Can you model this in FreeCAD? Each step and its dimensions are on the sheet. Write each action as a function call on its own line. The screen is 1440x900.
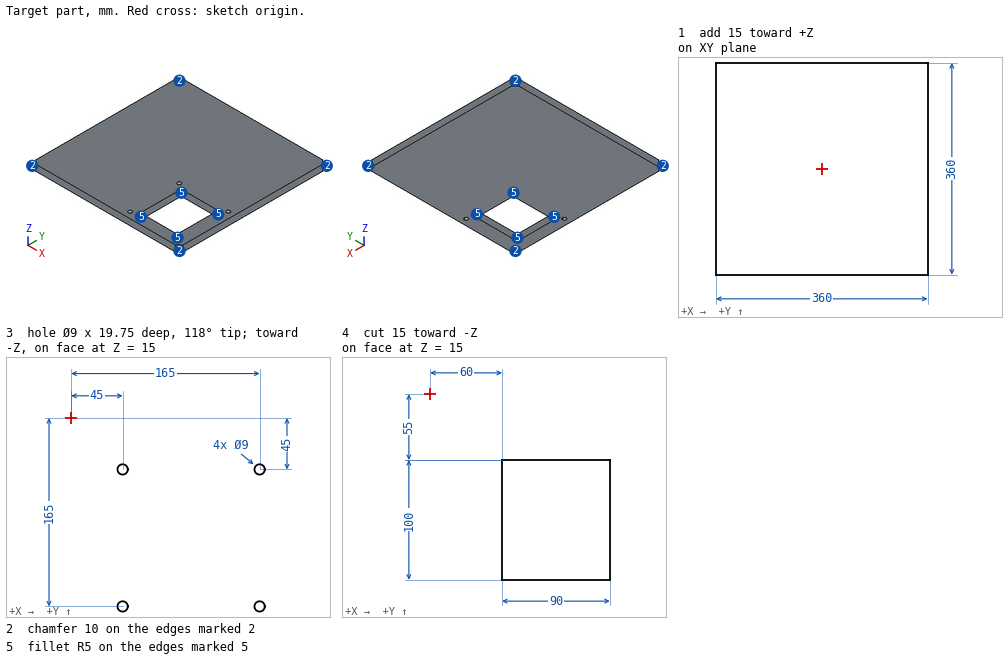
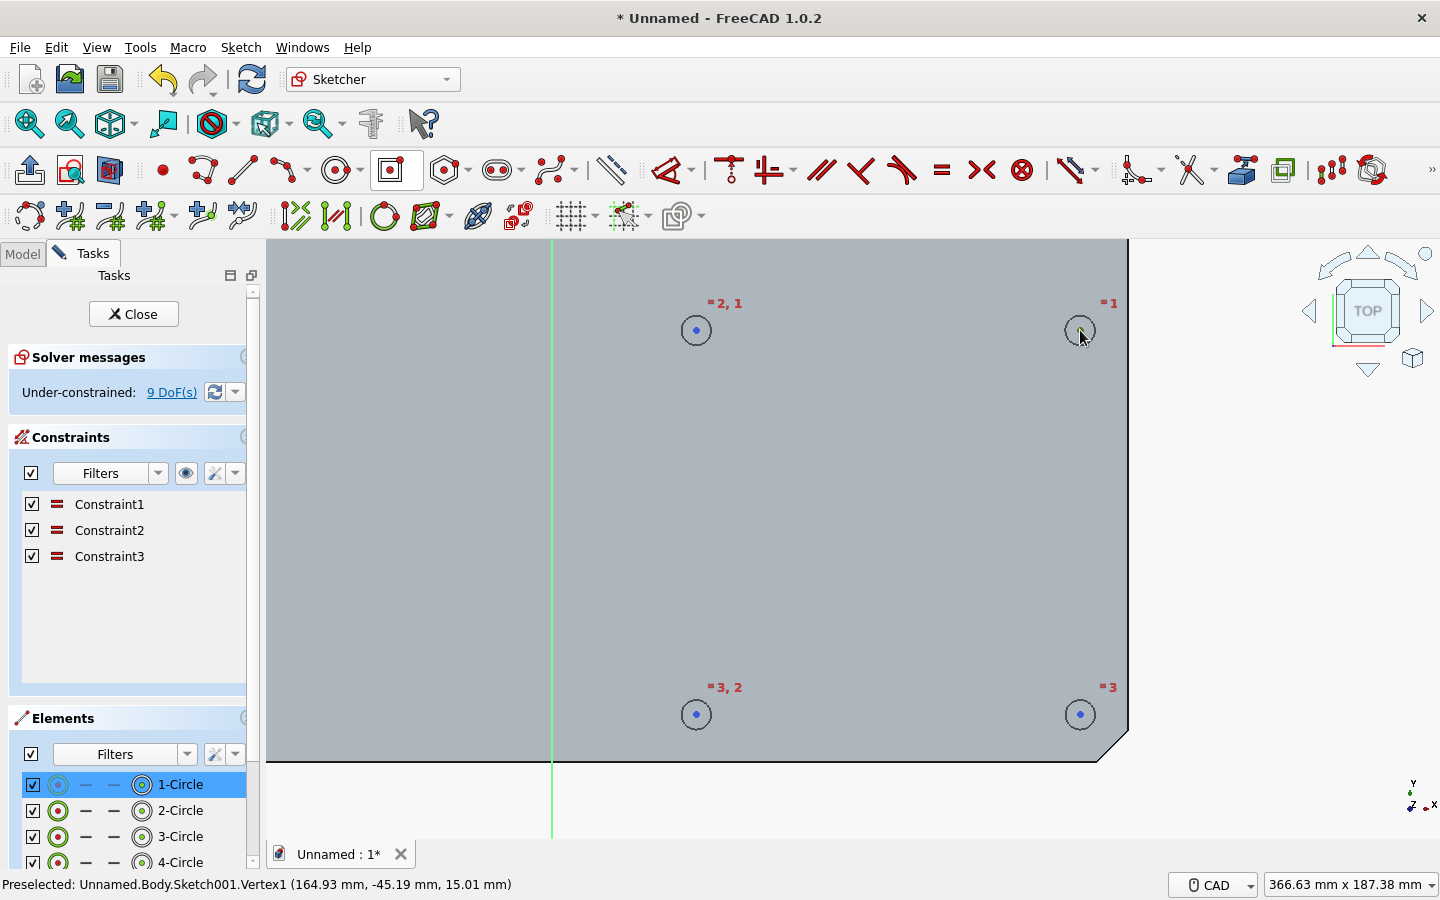
click(696, 330)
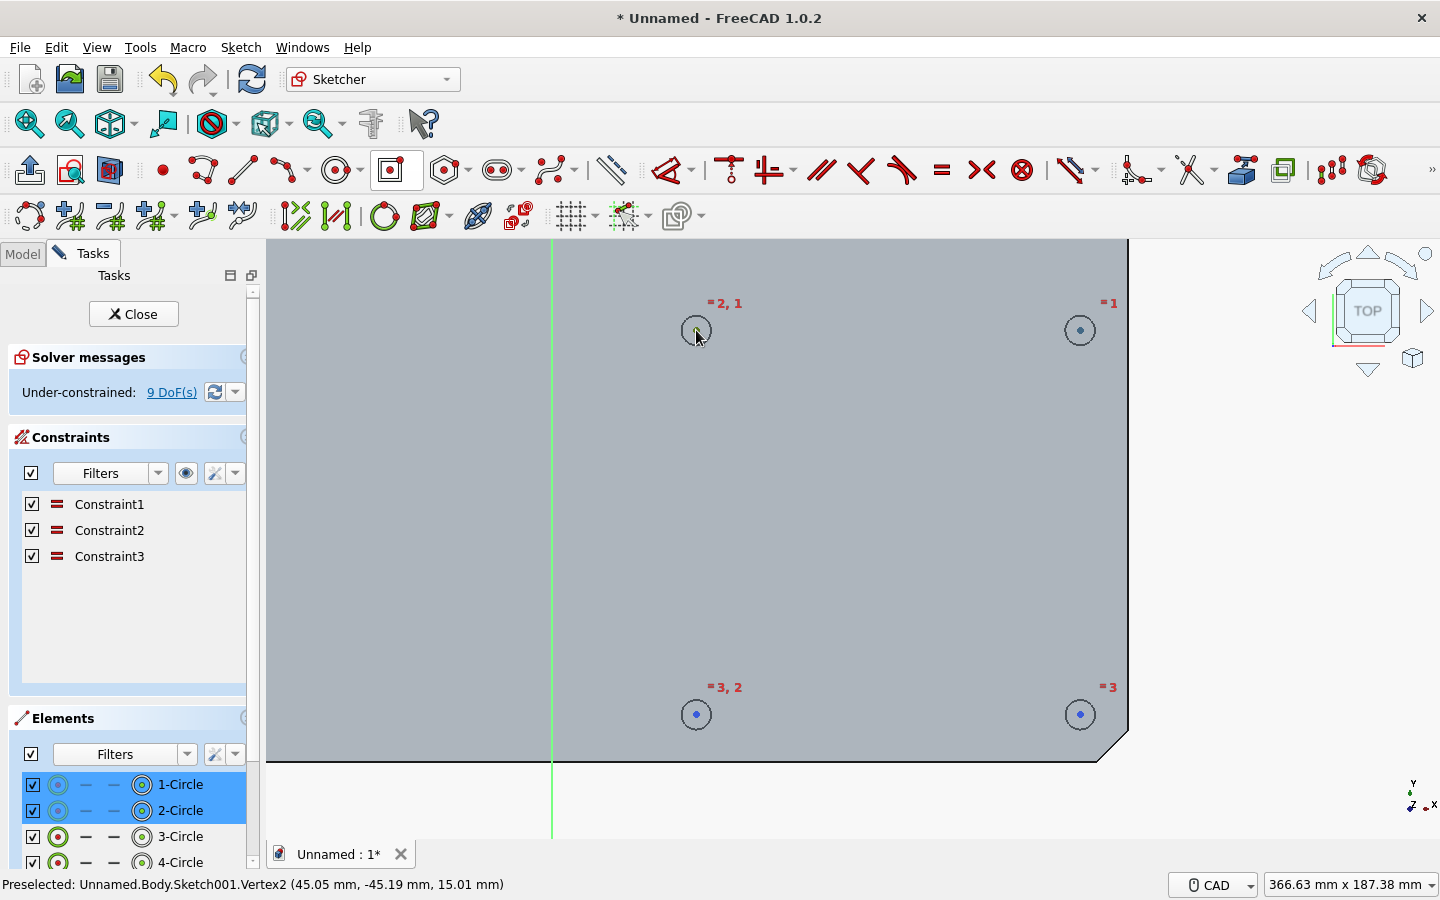
key(h)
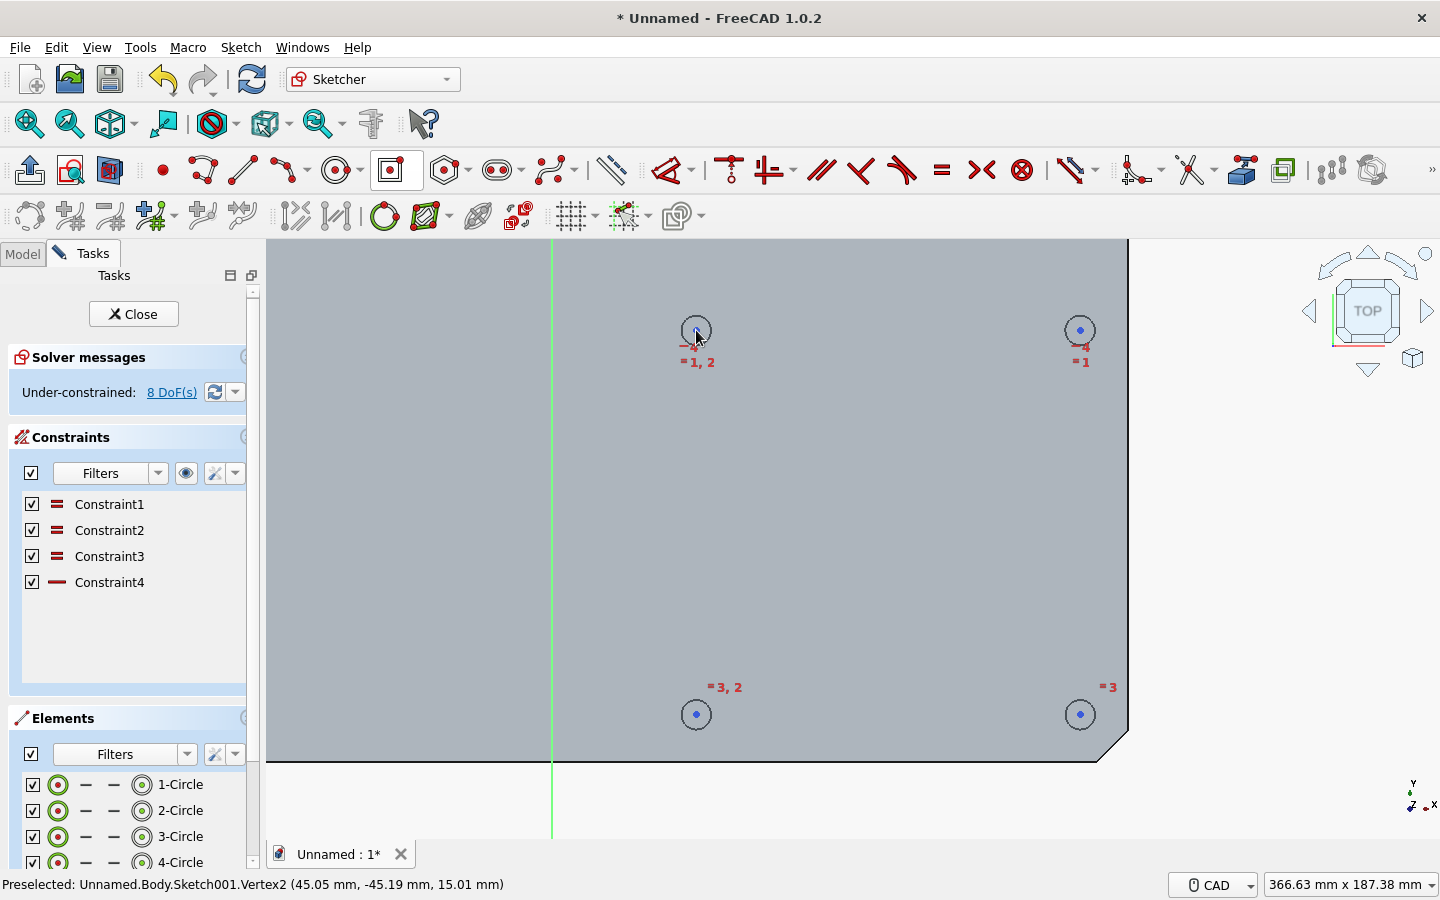
click(696, 330)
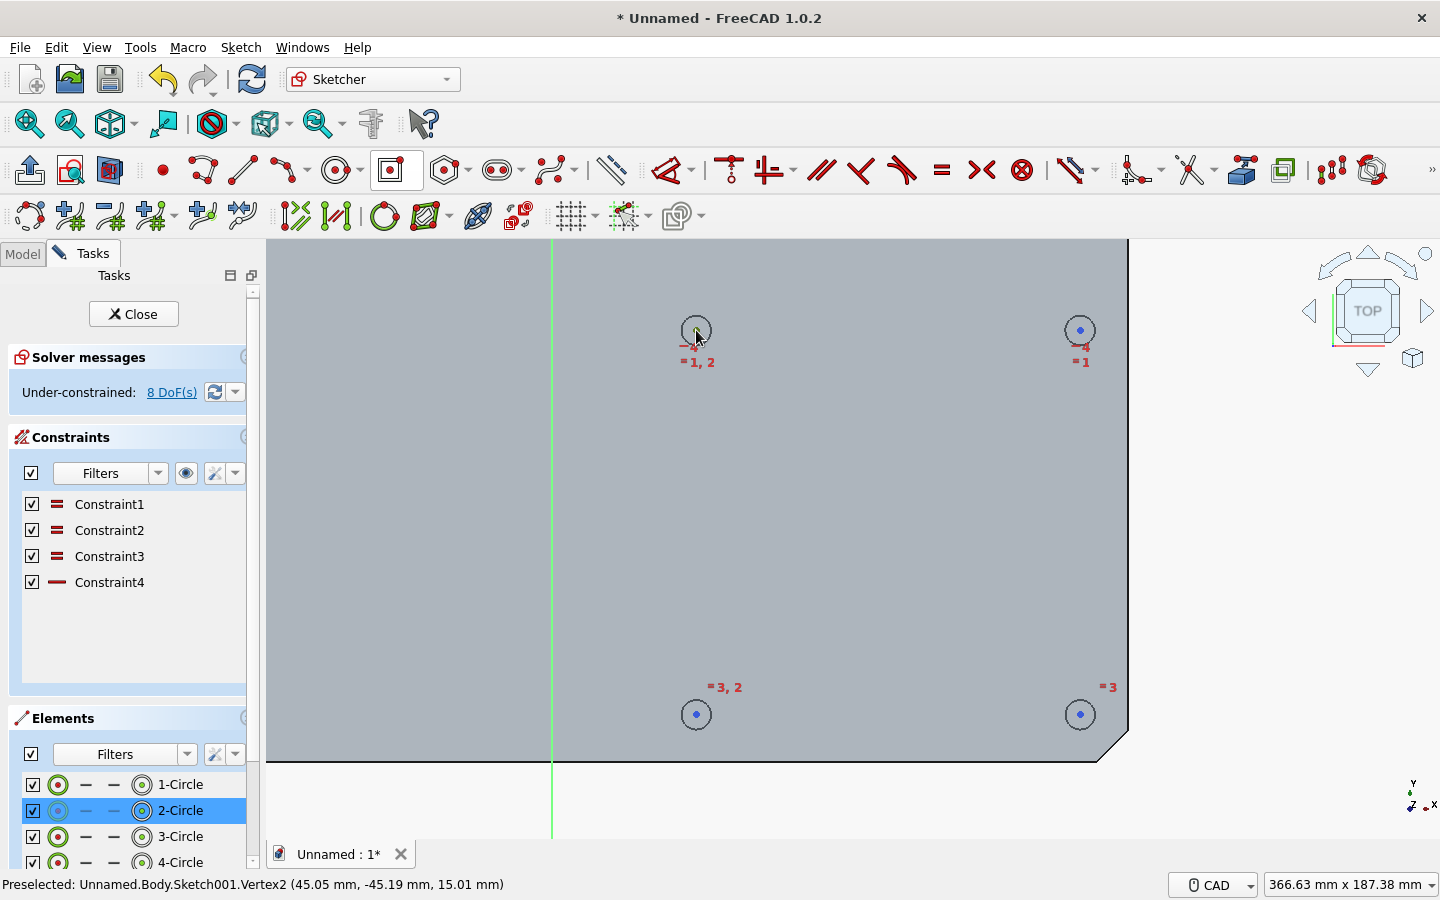
click(696, 715)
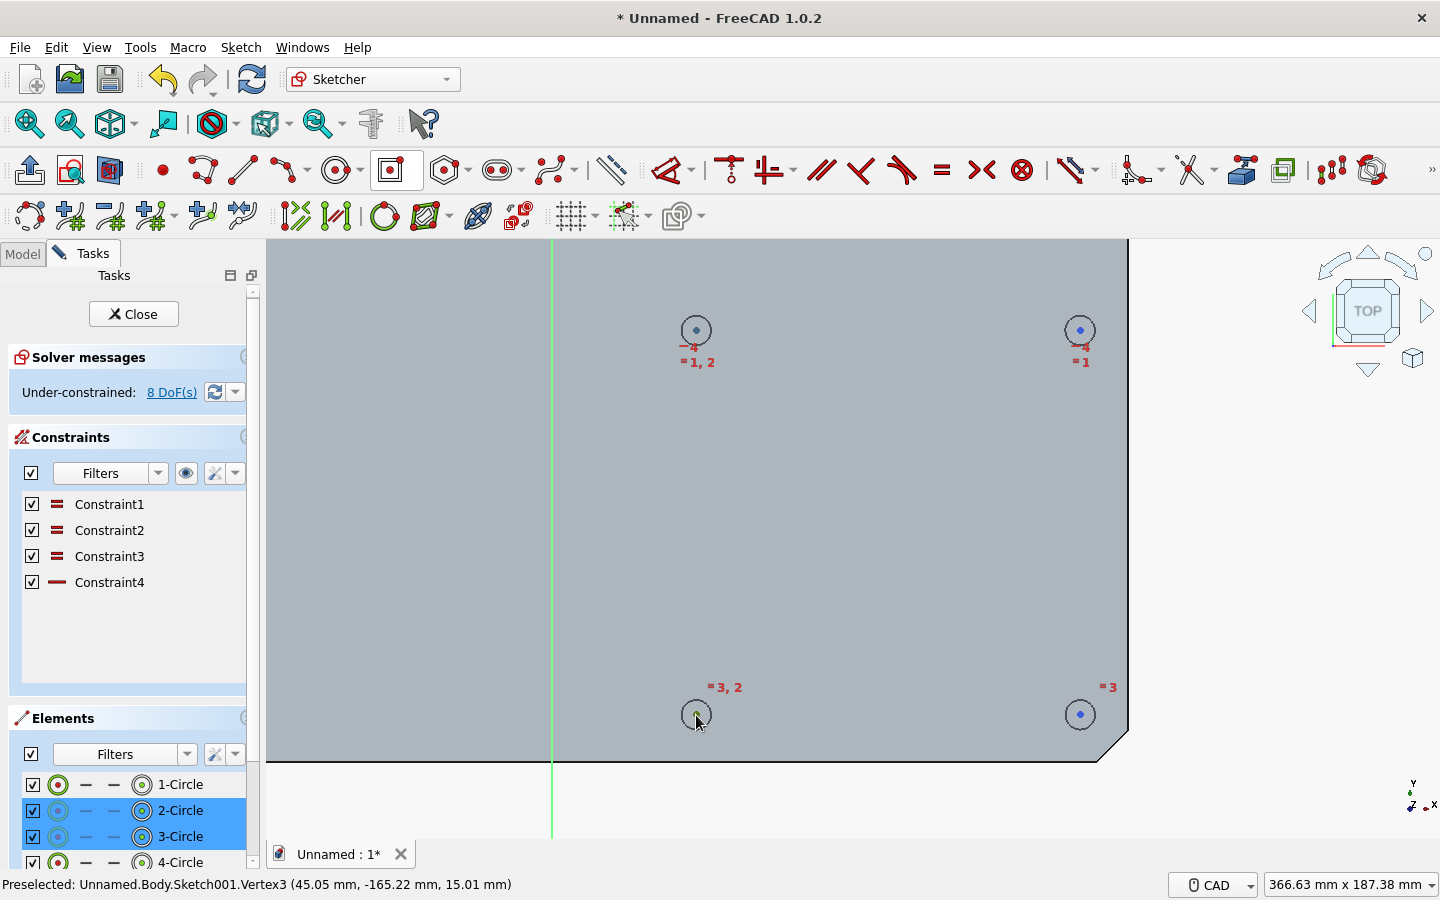
click(796, 170)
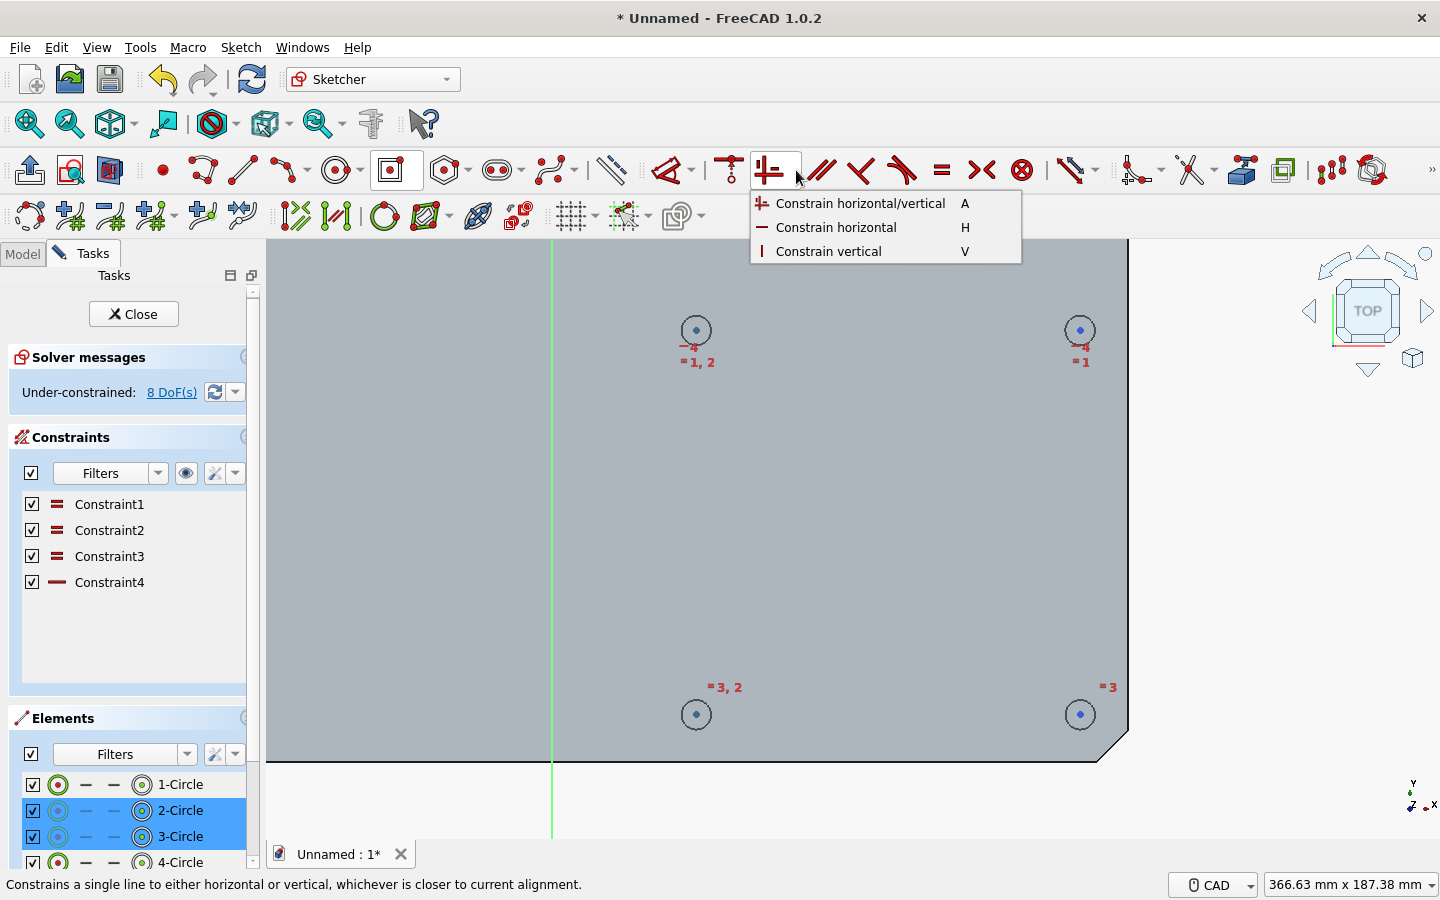
click(886, 251)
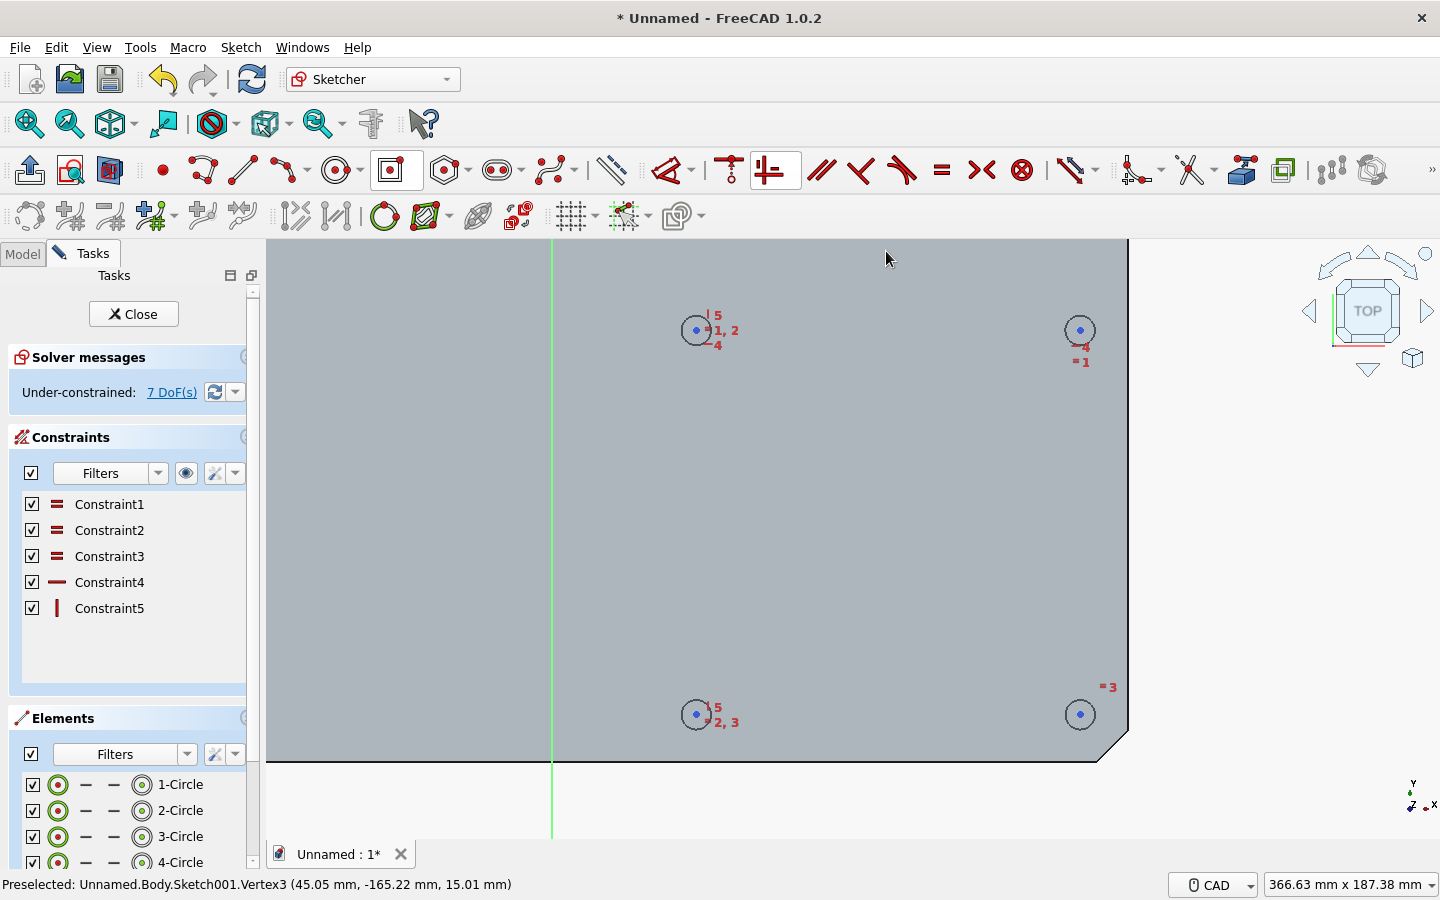
click(1080, 330)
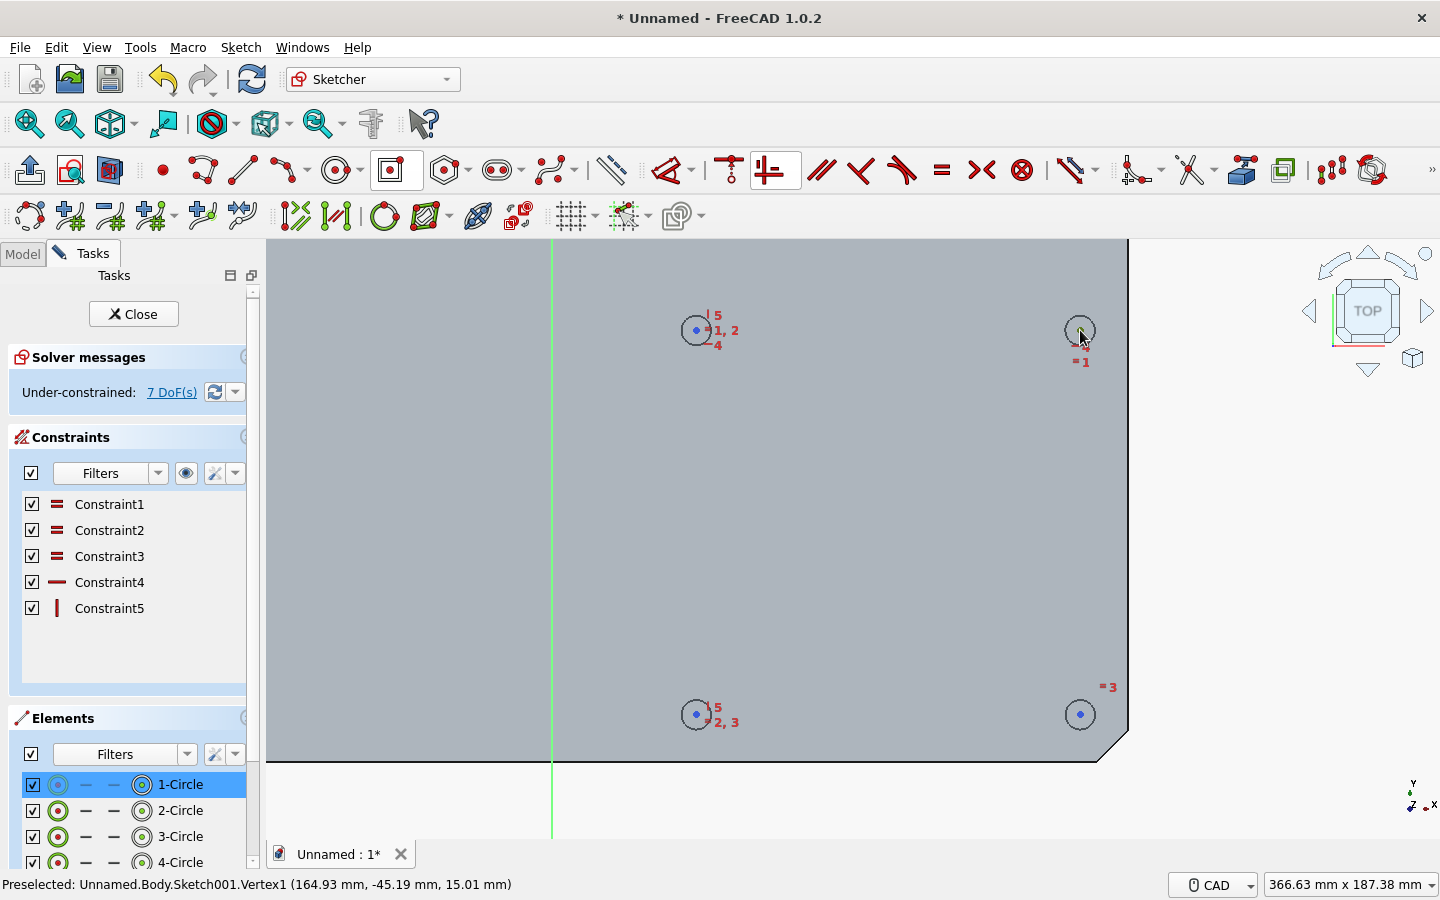
click(1080, 715)